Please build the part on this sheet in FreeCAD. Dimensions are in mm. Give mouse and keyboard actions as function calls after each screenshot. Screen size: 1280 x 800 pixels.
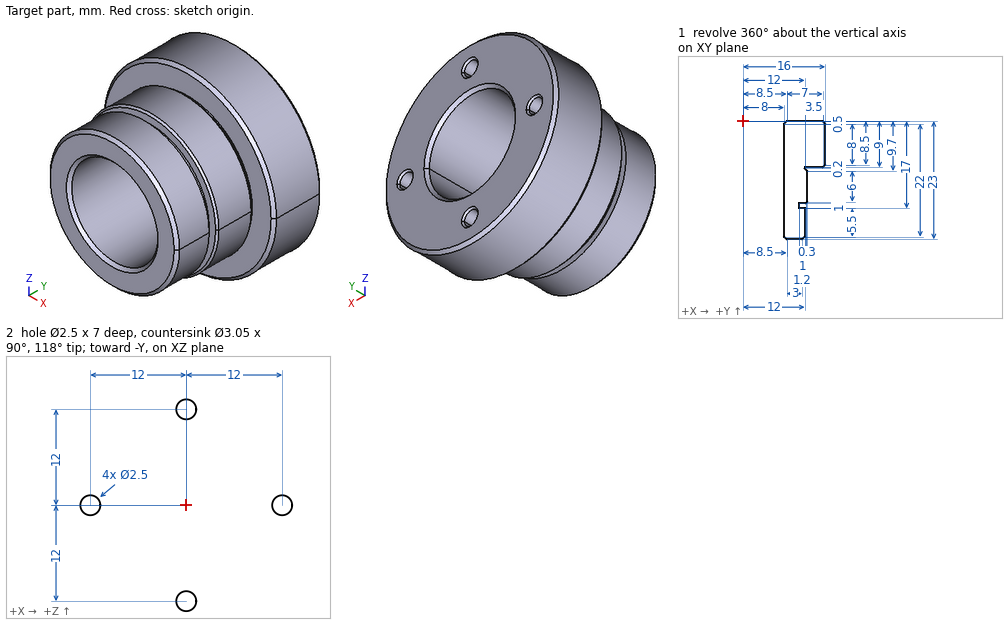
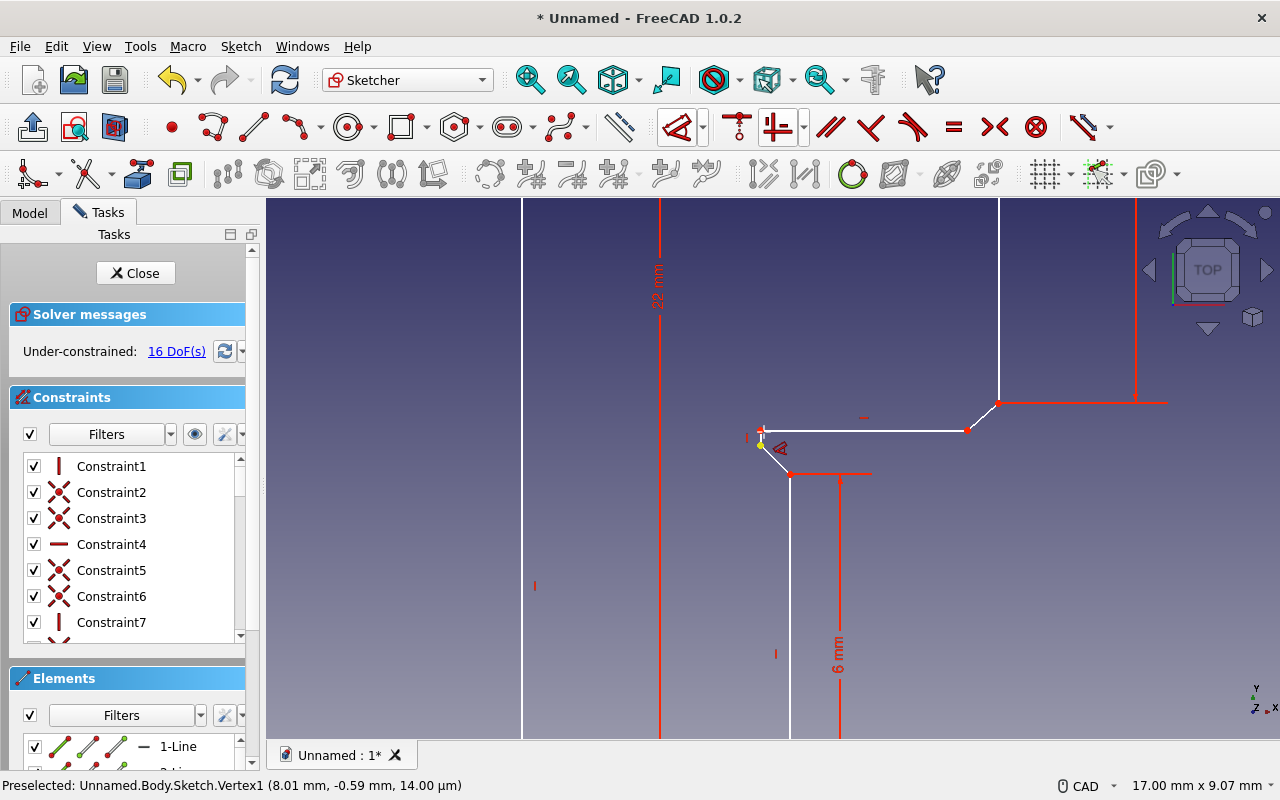
click(761, 431)
click(795, 328)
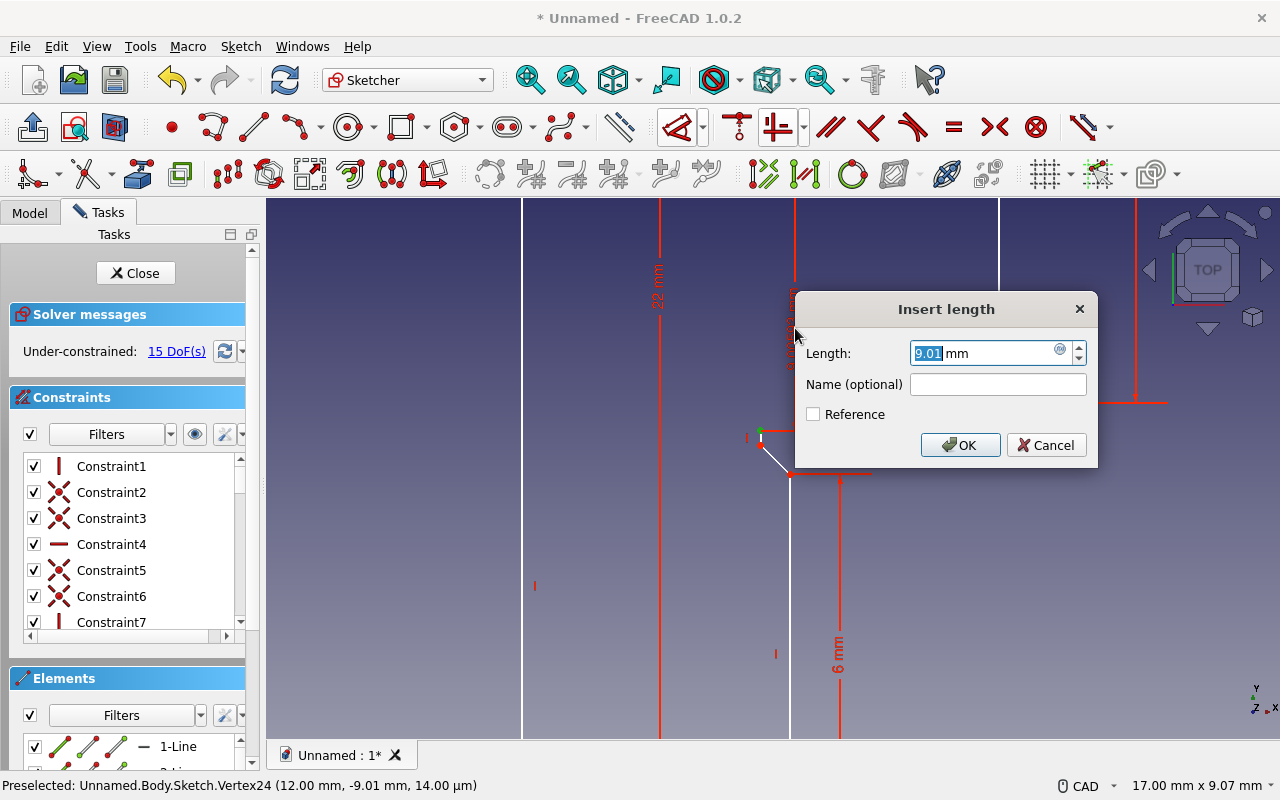
text(9)
key(Return)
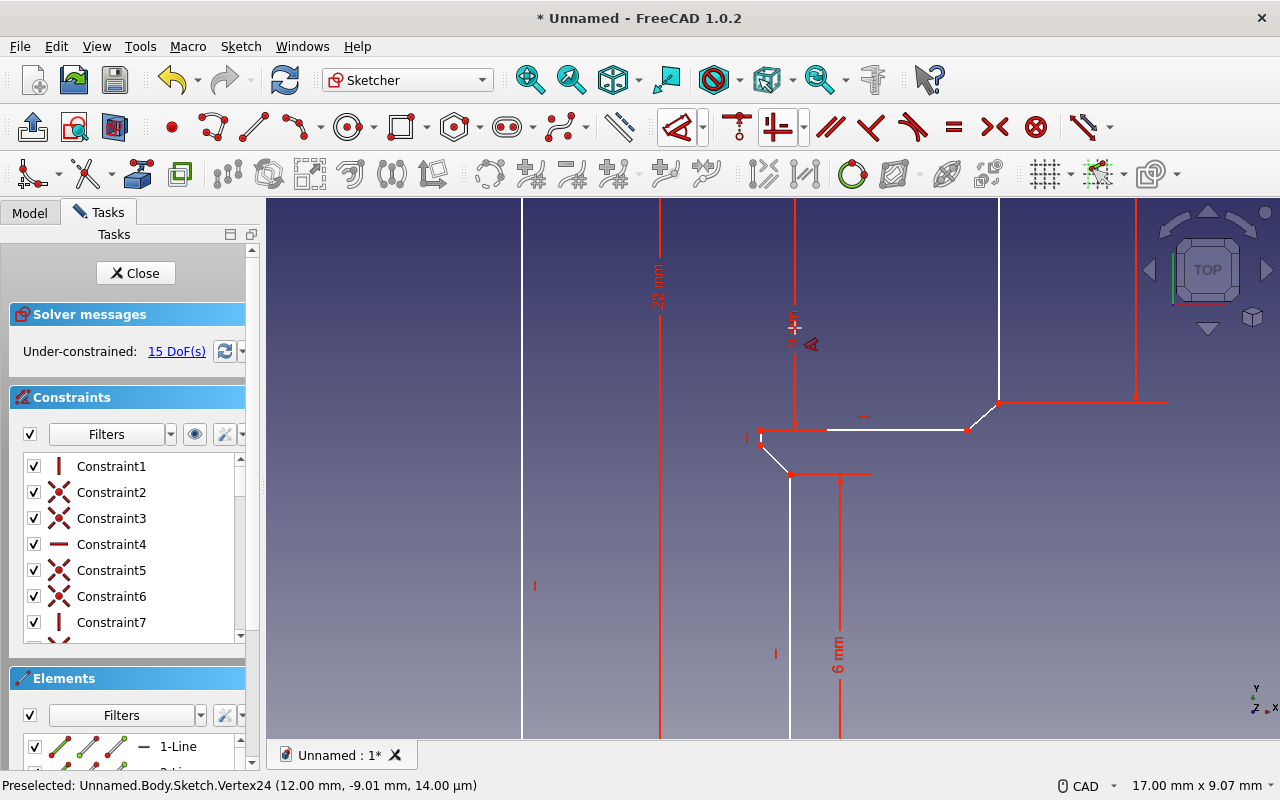
scroll(764, 432, down, 7)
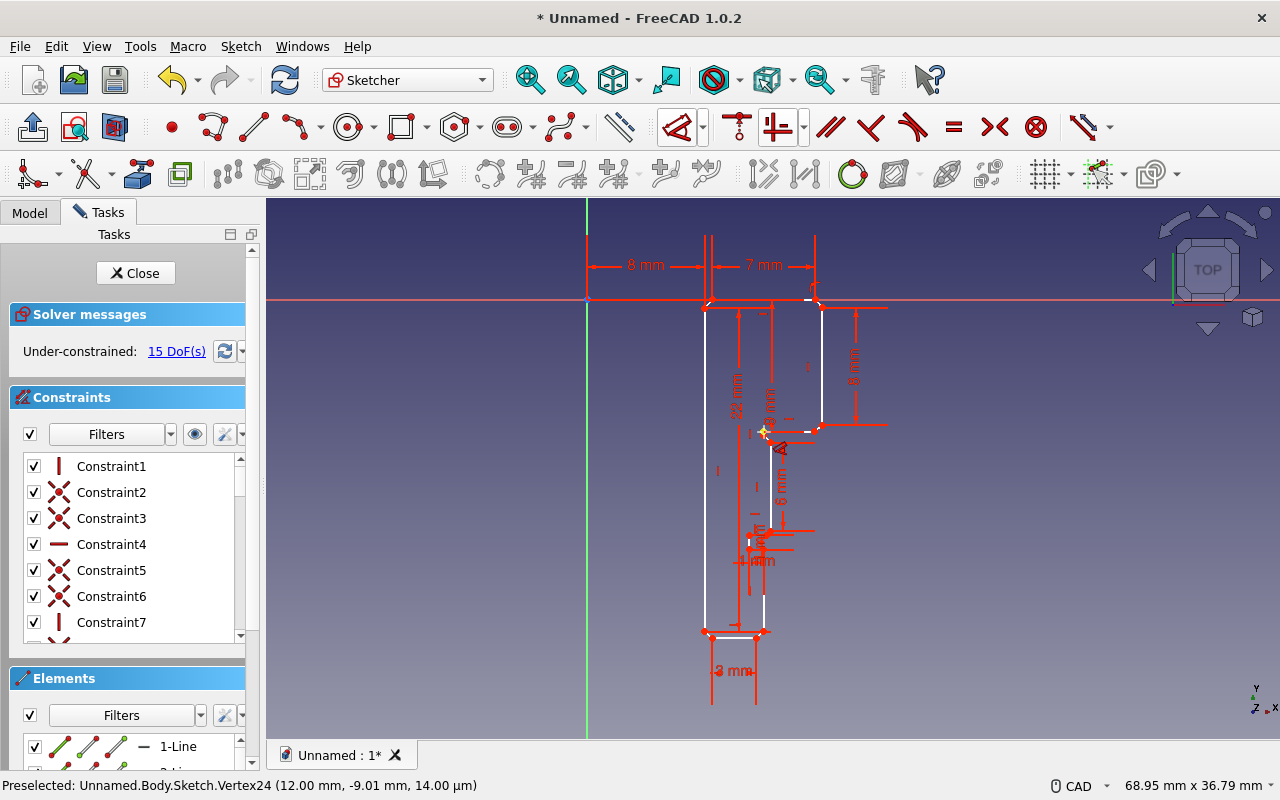
click(764, 607)
click(798, 590)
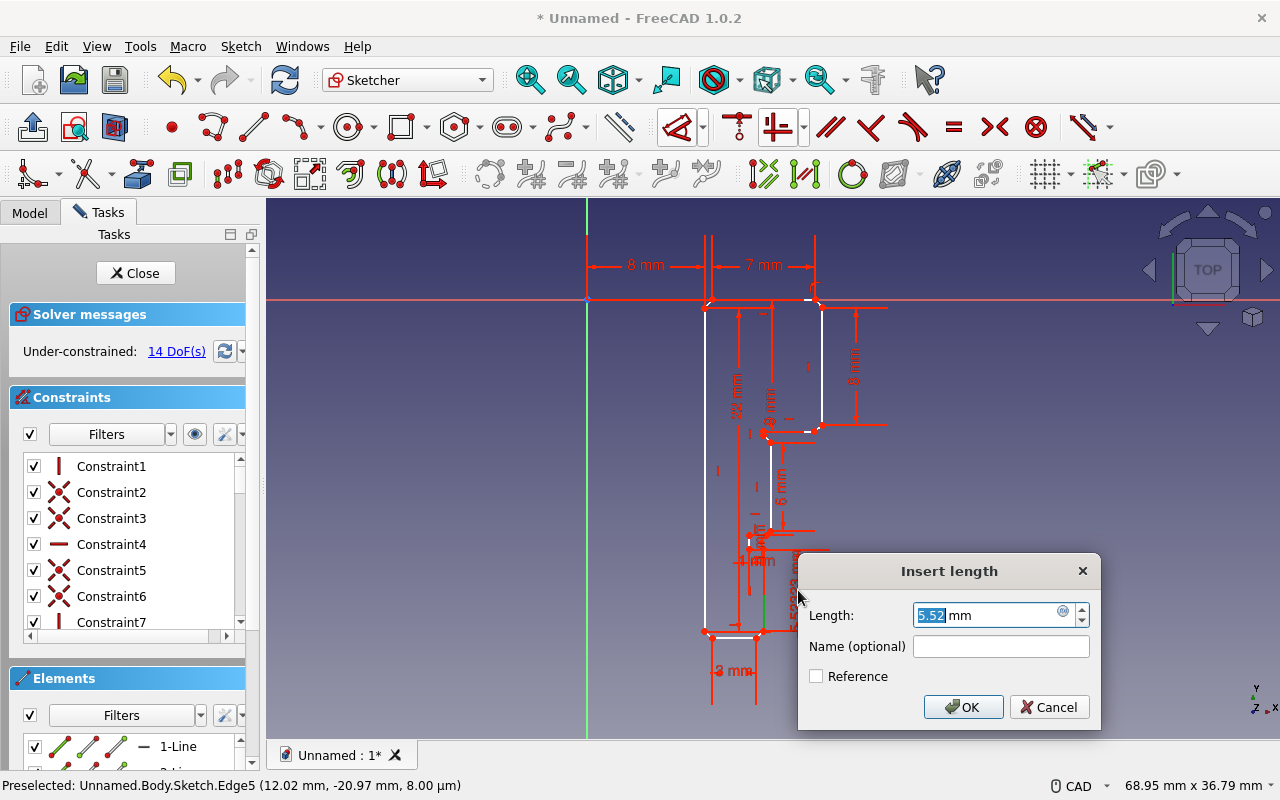
text(5.5)
key(Return)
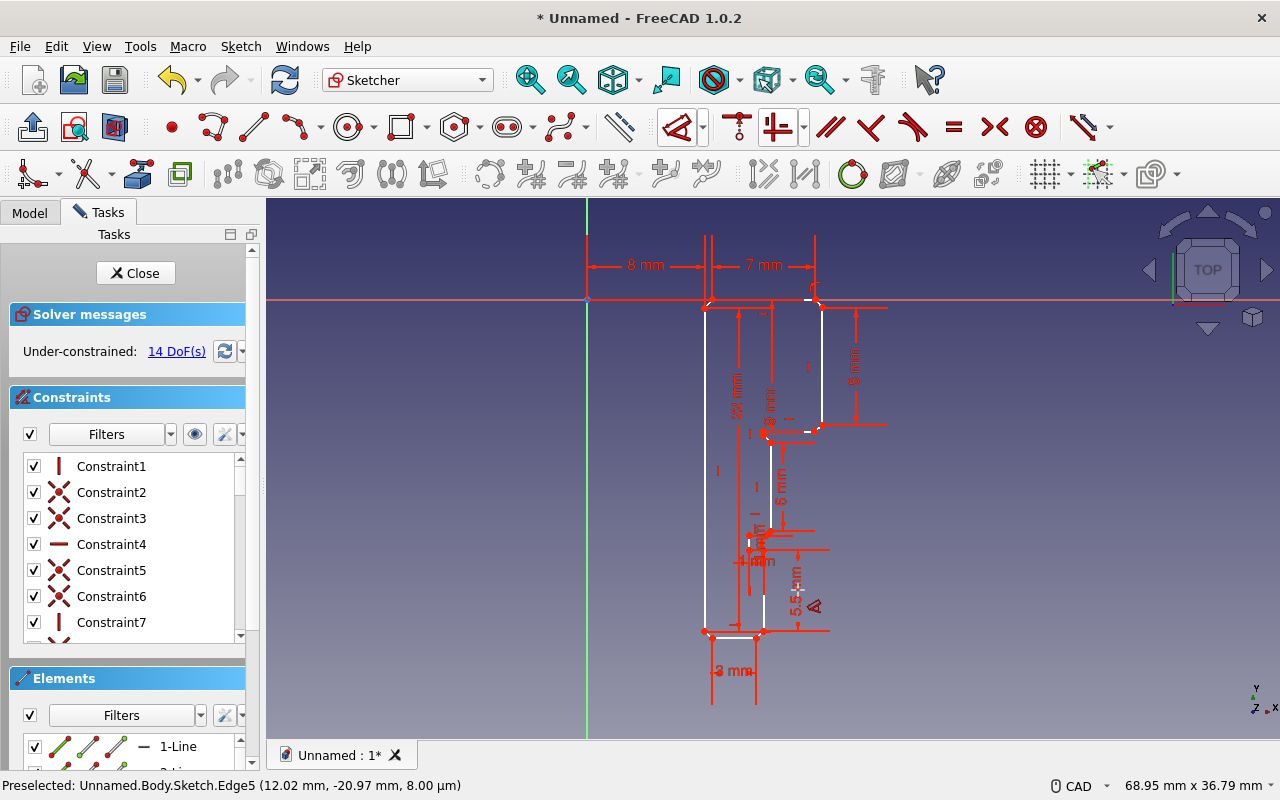
scroll(758, 536, up, 5)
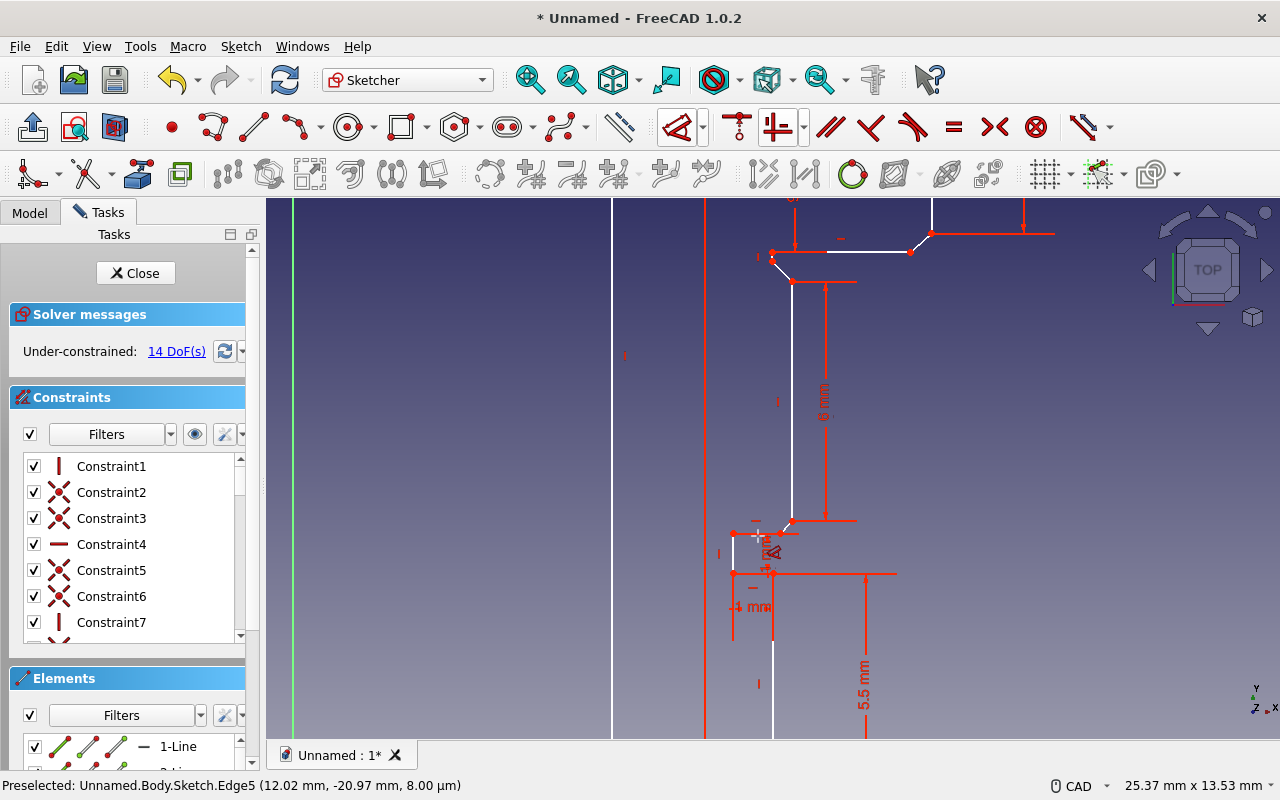
click(757, 534)
click(757, 500)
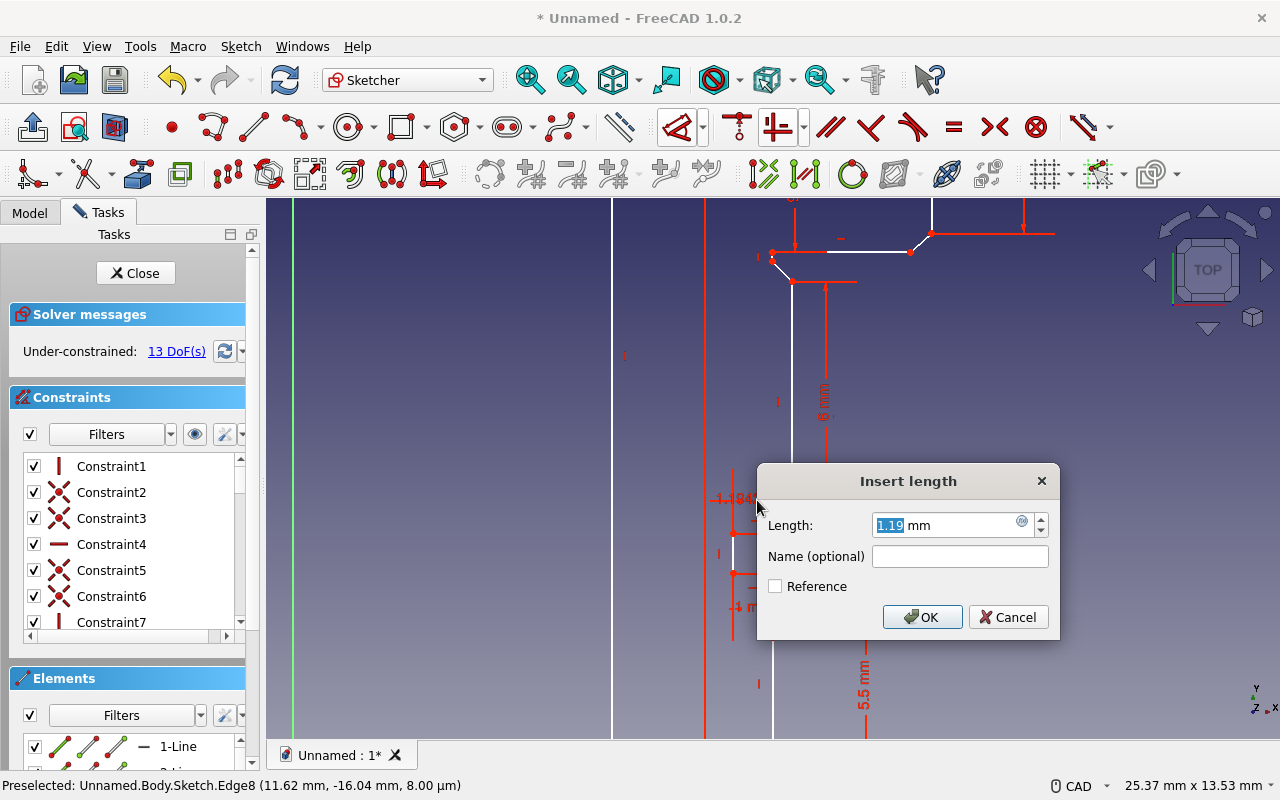
text(1.2)
key(Return)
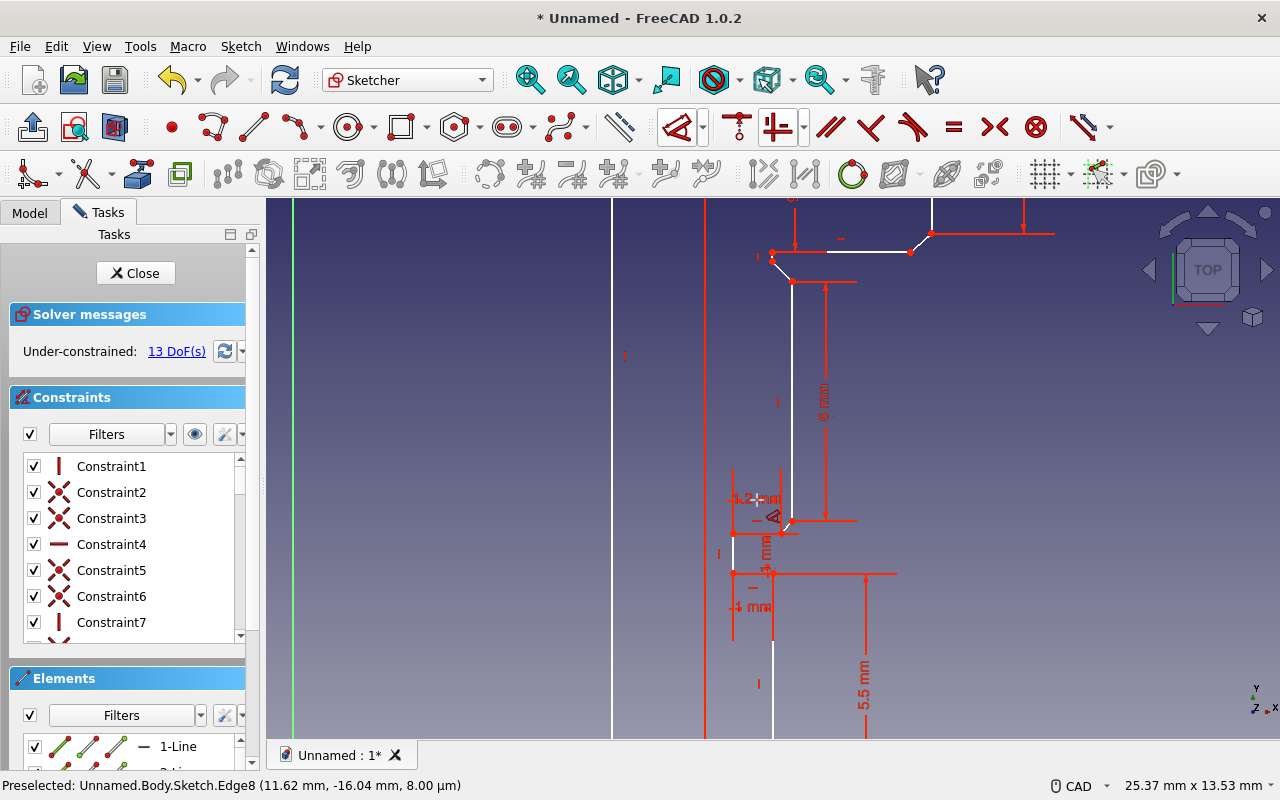
scroll(772, 257, up, 9)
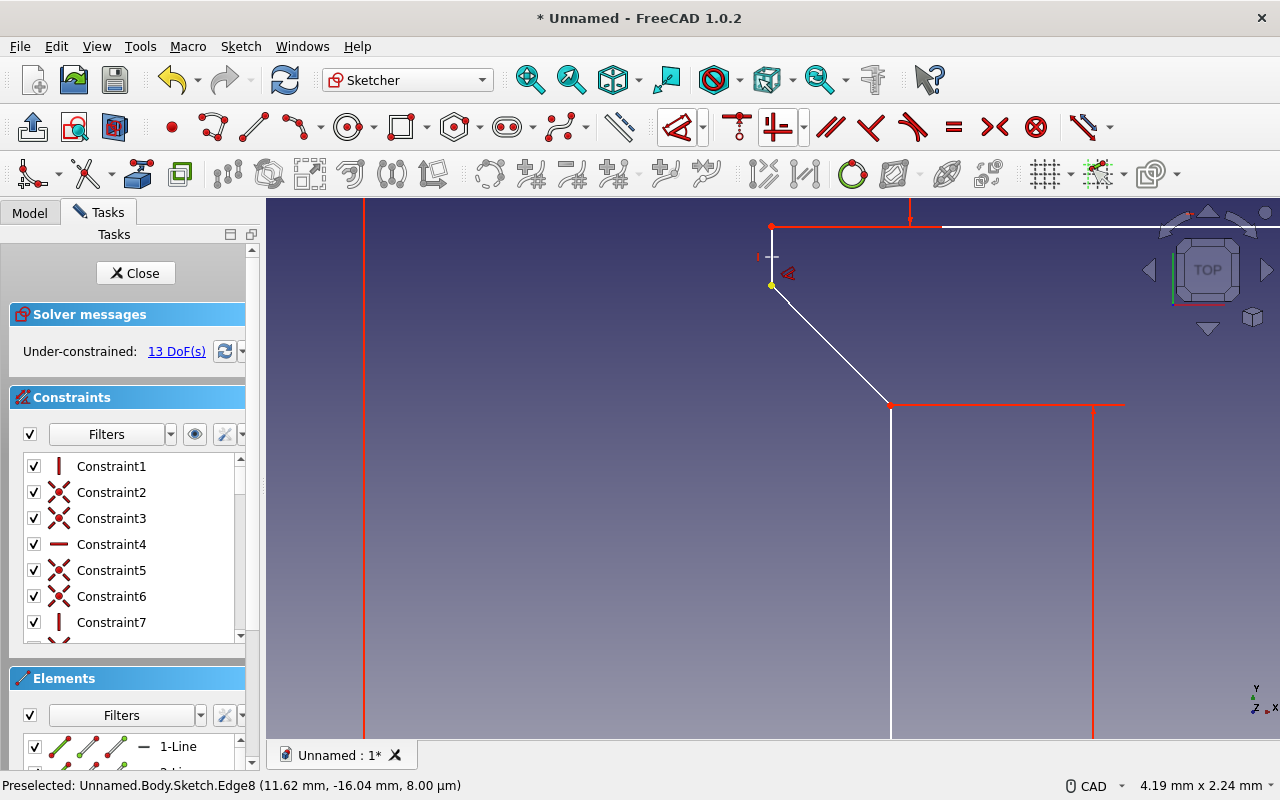
click(772, 256)
click(806, 256)